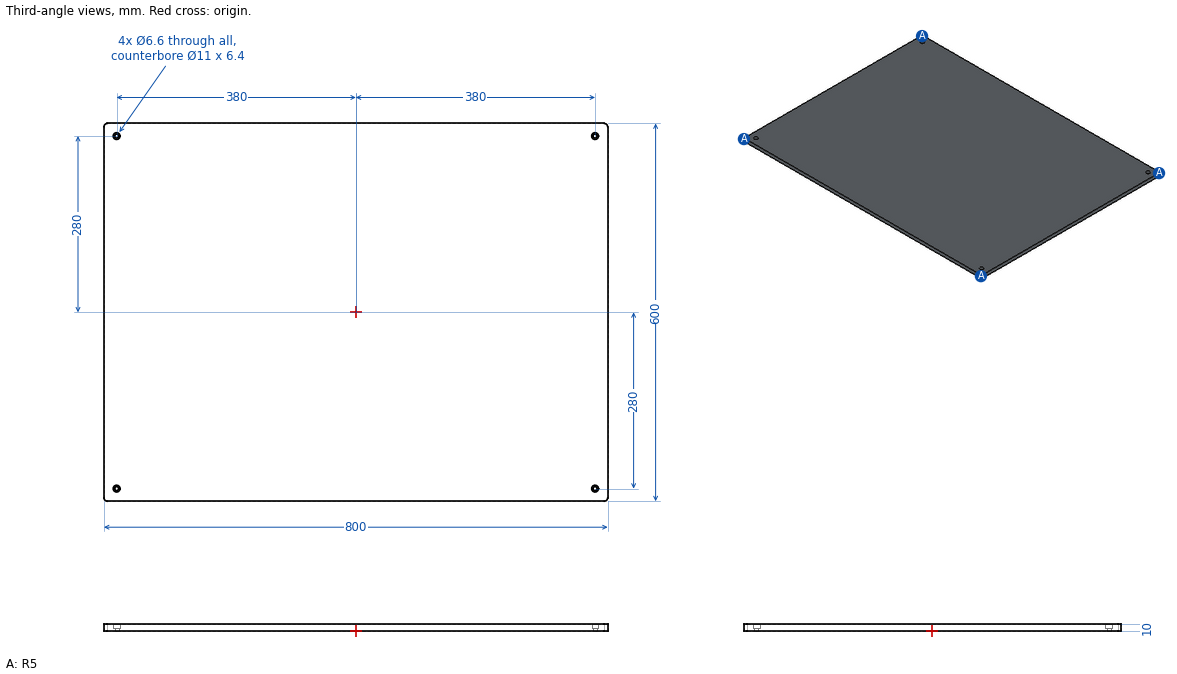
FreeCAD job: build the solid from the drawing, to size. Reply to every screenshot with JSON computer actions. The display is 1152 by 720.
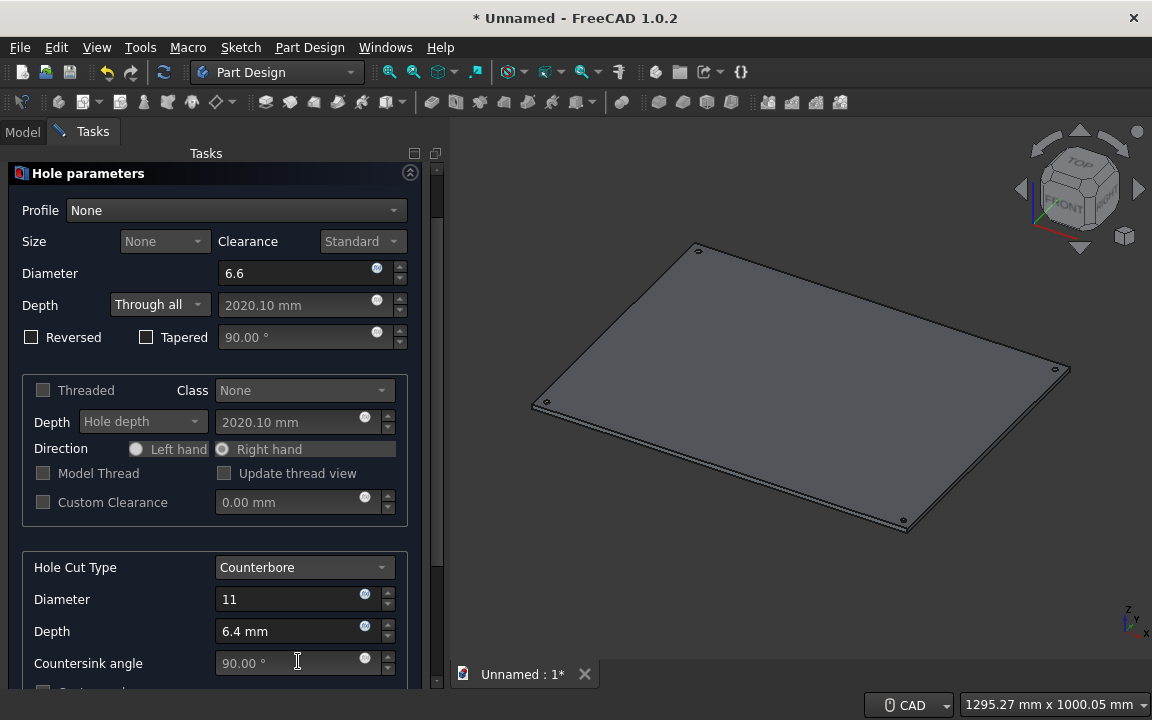
{"action": "scroll", "coordinate": [437, 426], "scroll_direction": "up", "scroll_amount": 2}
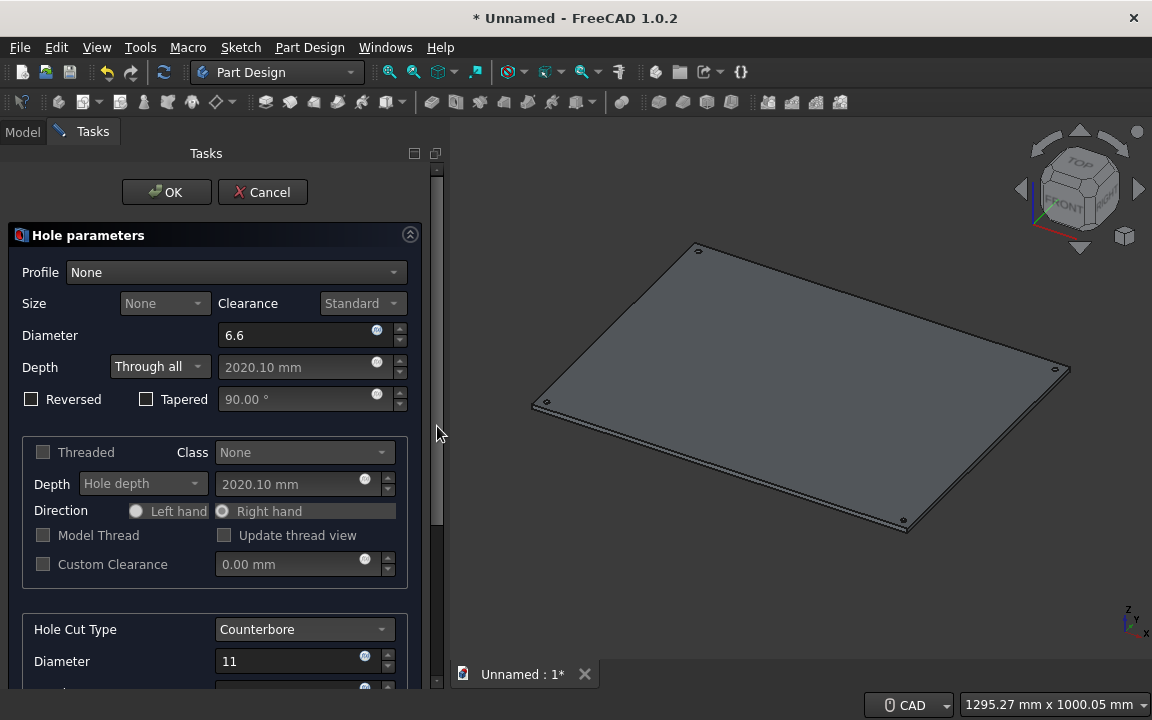
{"action": "left_click", "coordinate": [167, 192]}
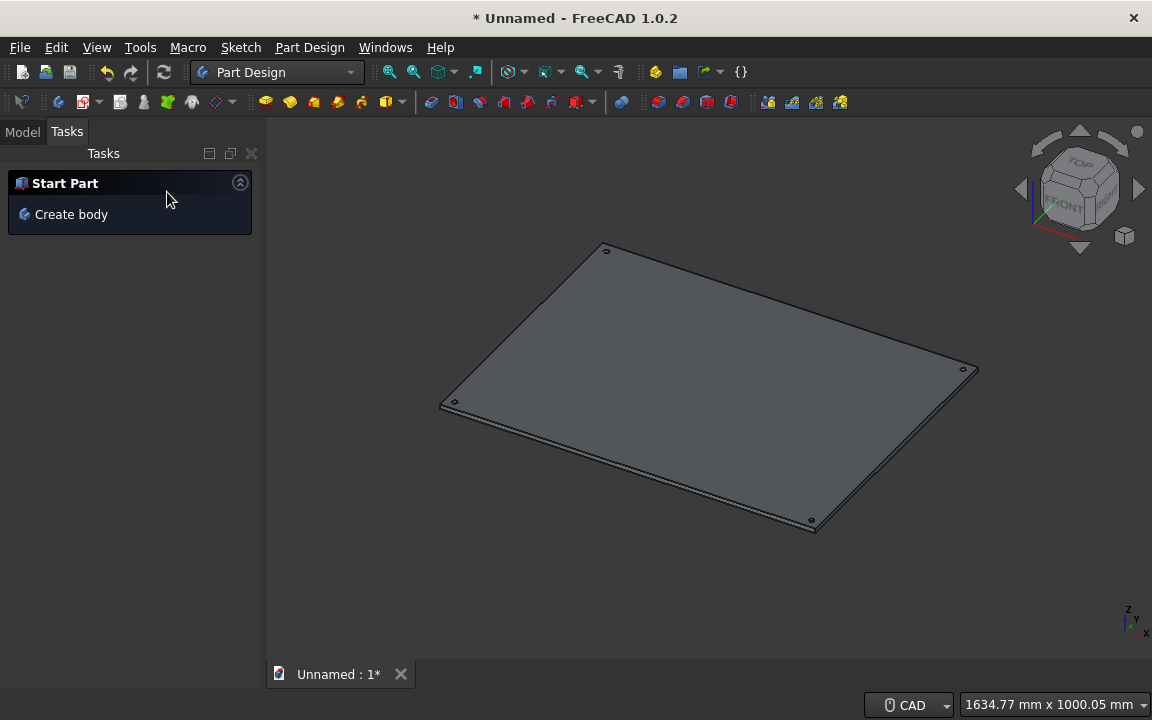
{"action": "scroll", "coordinate": [815, 530], "scroll_direction": "up", "scroll_amount": 10}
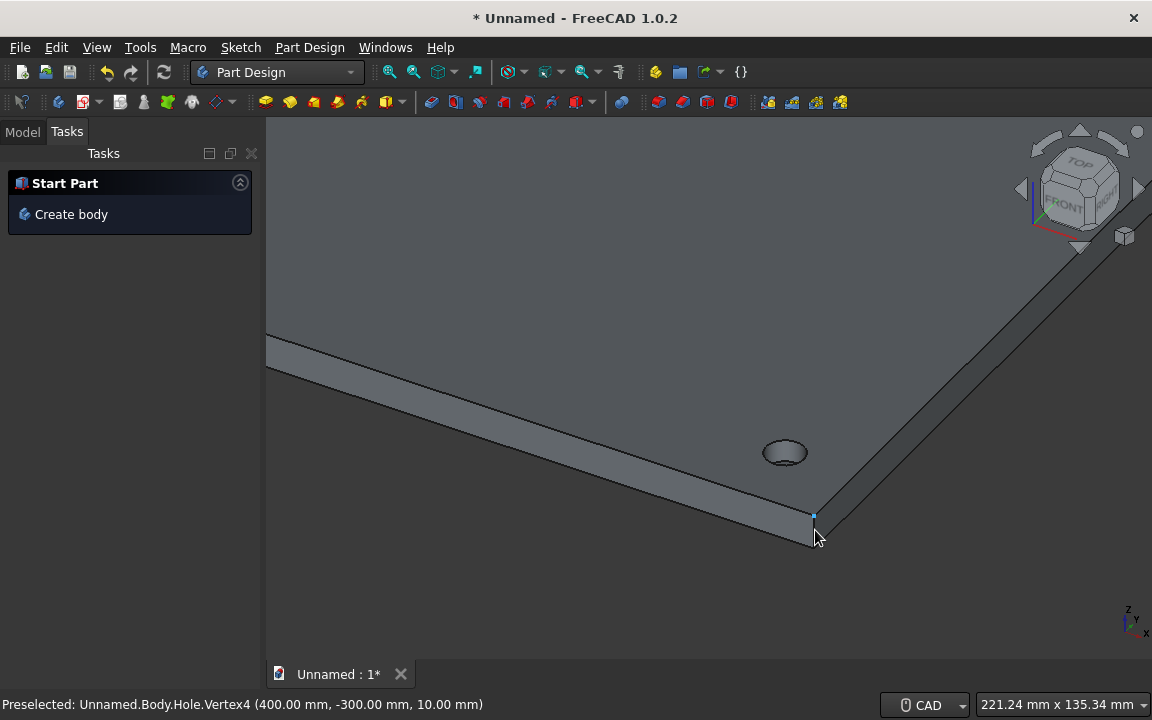
{"action": "left_click", "coordinate": [814, 531]}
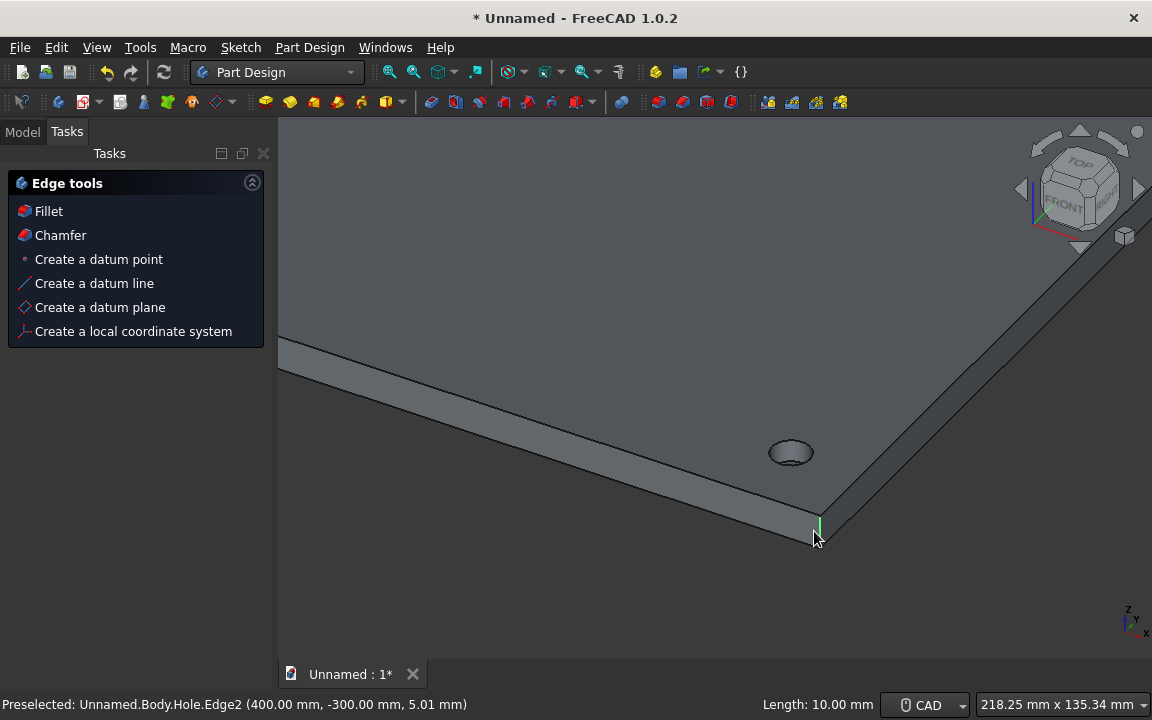
{"action": "left_click", "coordinate": [390, 72]}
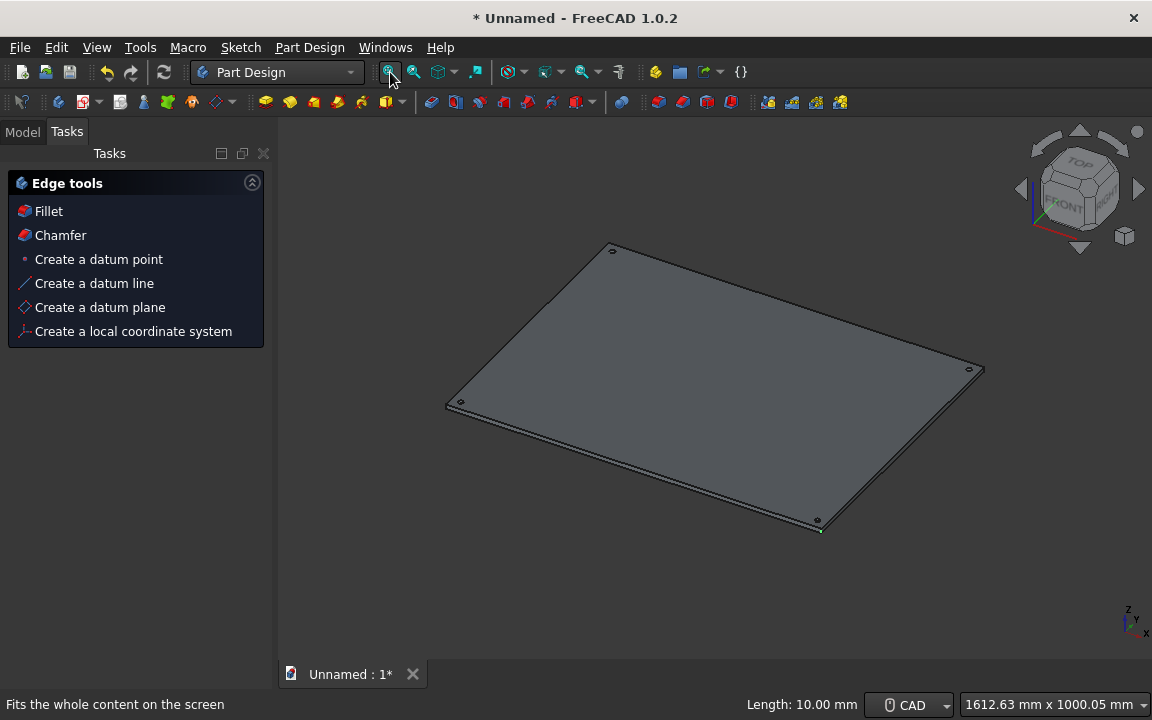
{"action": "key", "text": "0"}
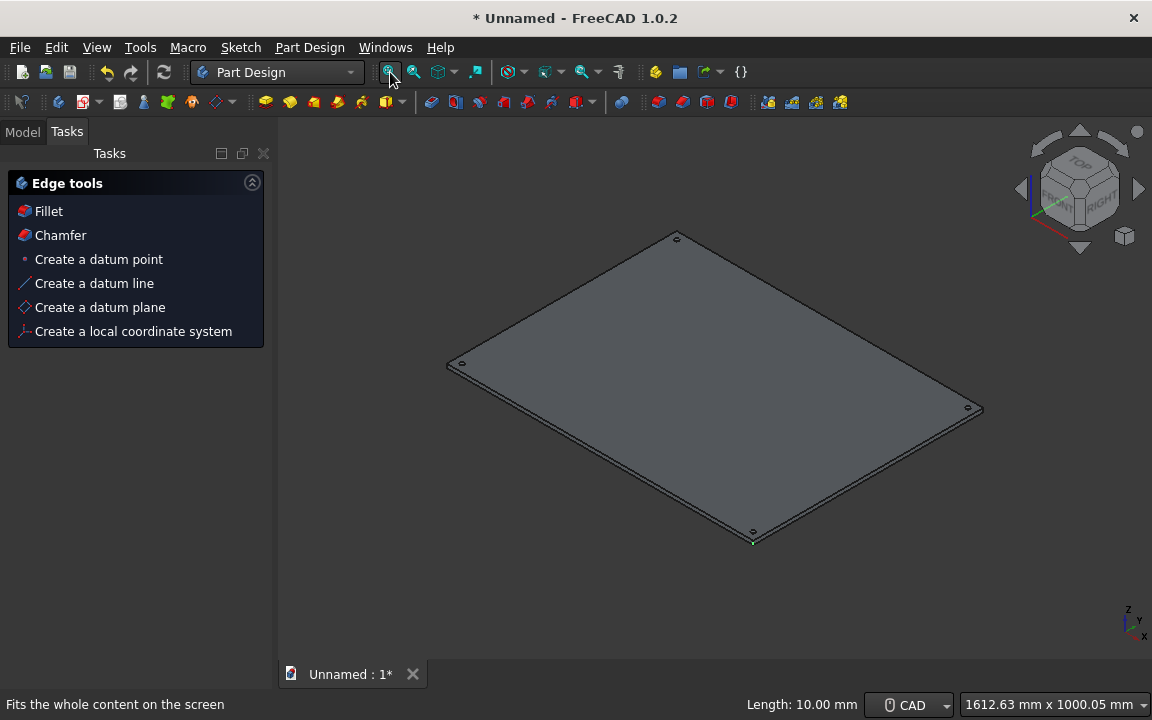
{"action": "scroll", "coordinate": [447, 365], "scroll_direction": "up", "scroll_amount": 10}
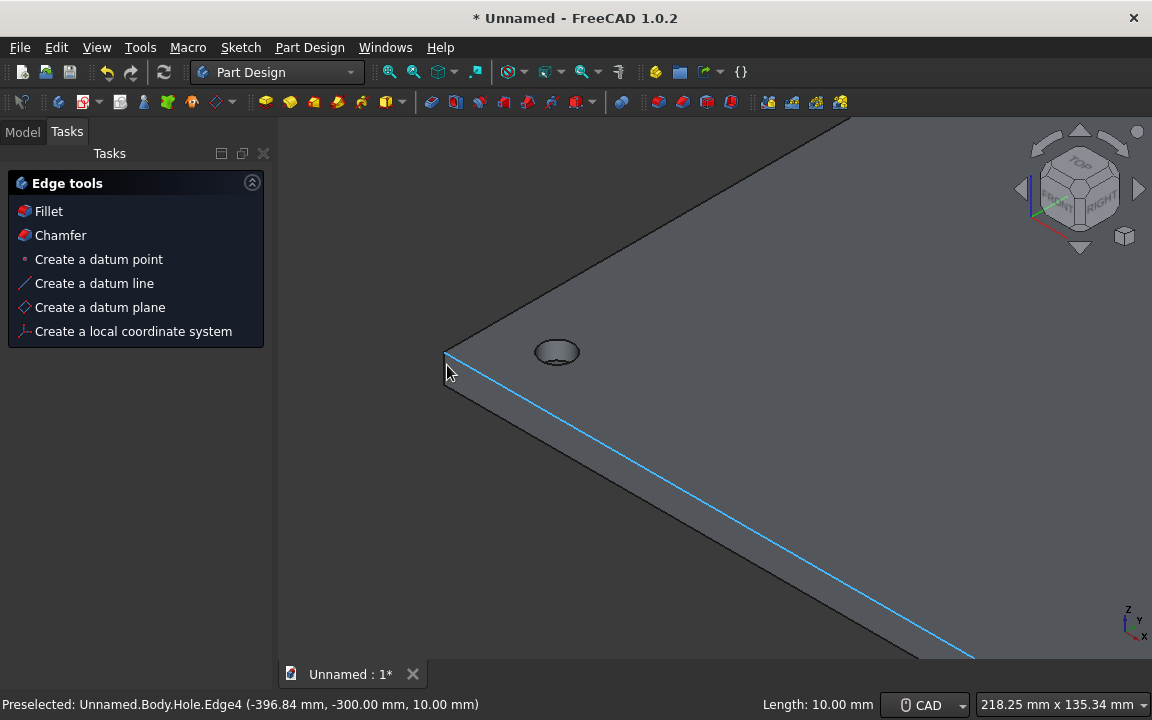
{"action": "key", "text": "v f"}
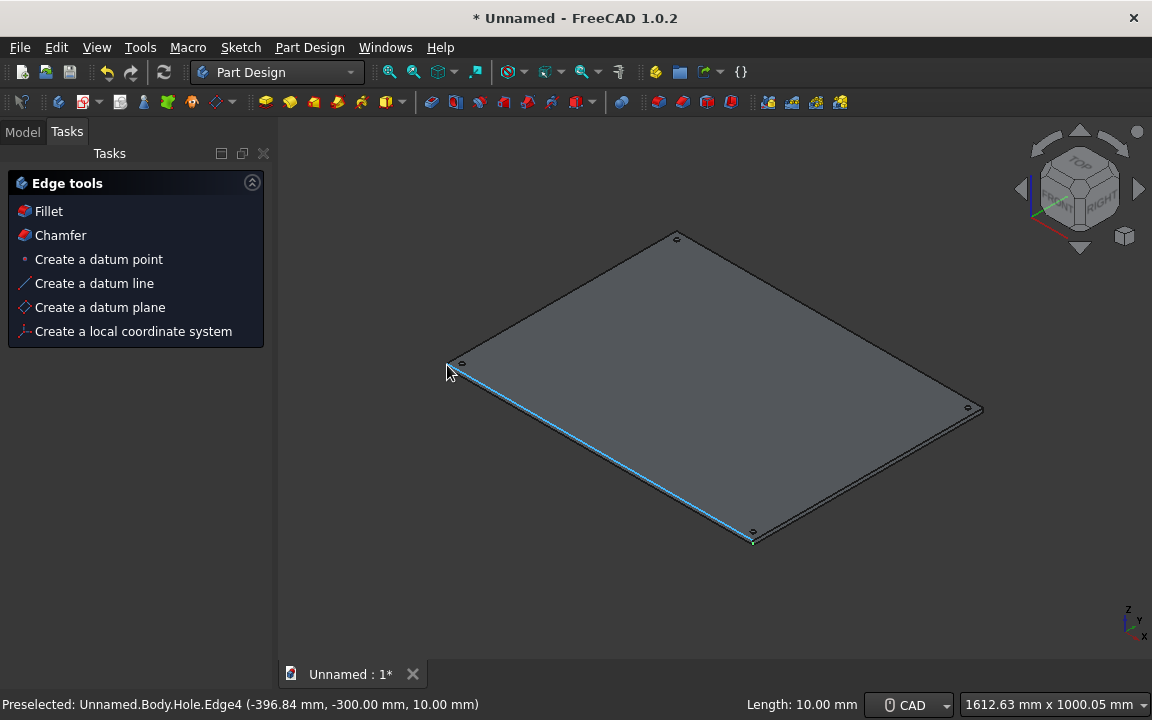
{"action": "key", "text": "2"}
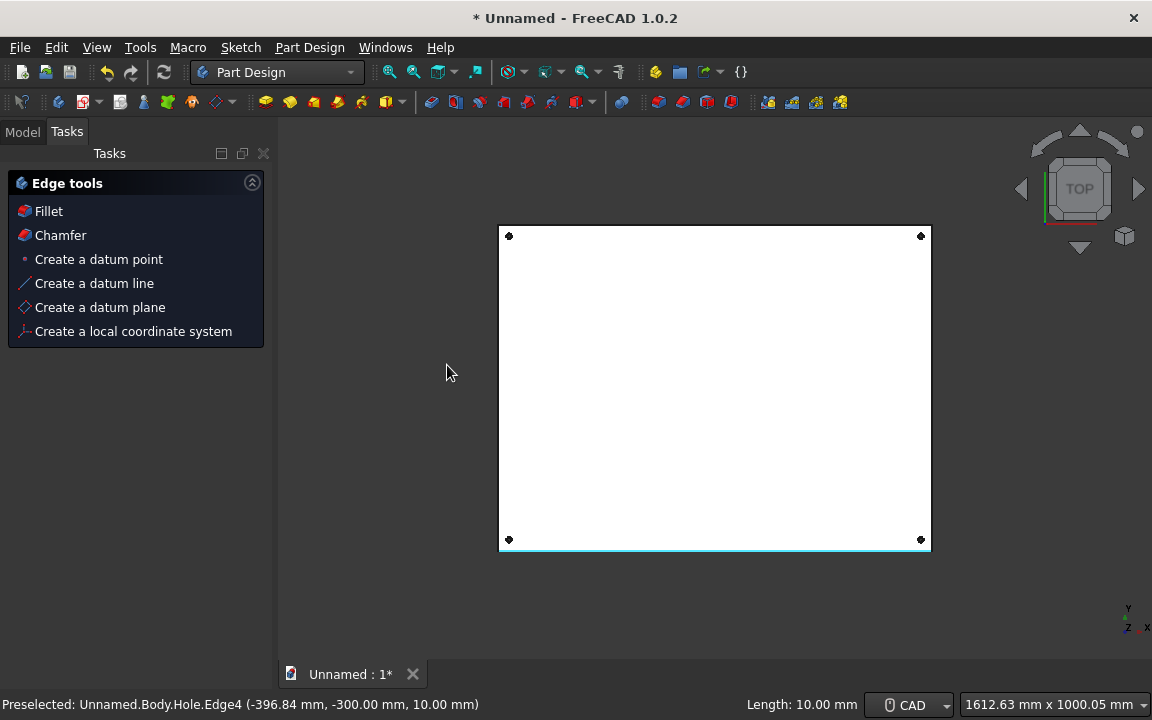
{"action": "scroll", "coordinate": [498, 550], "scroll_direction": "up", "scroll_amount": 10}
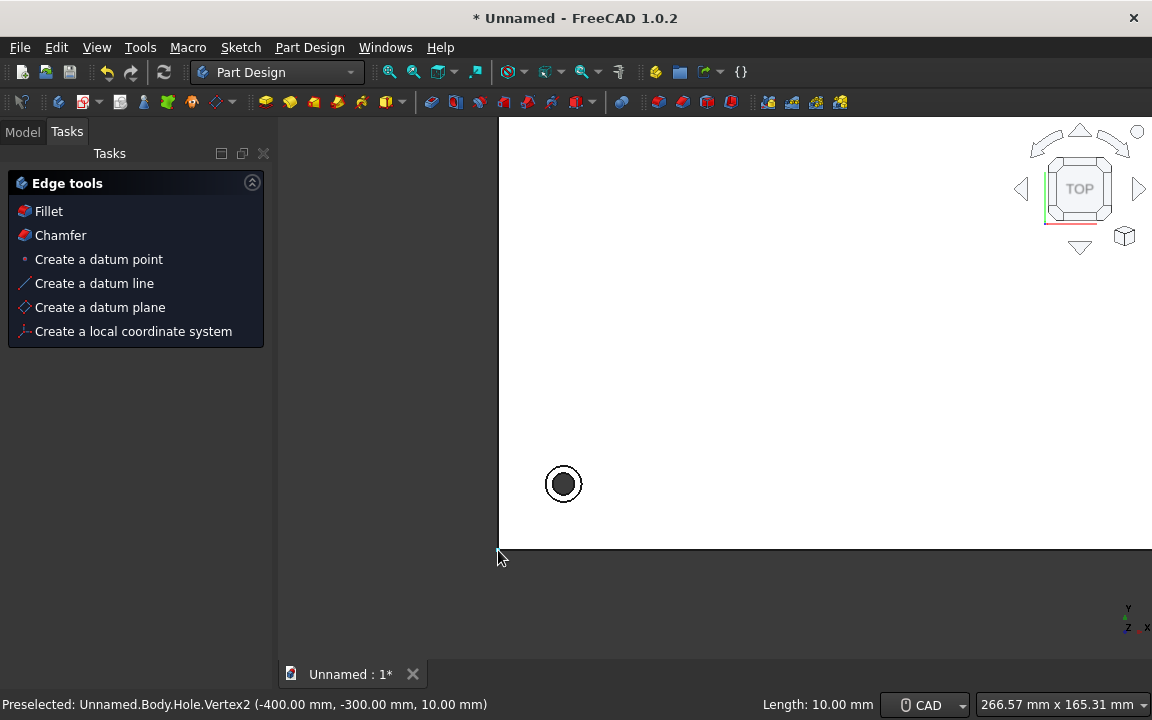
{"action": "key", "text": "v f"}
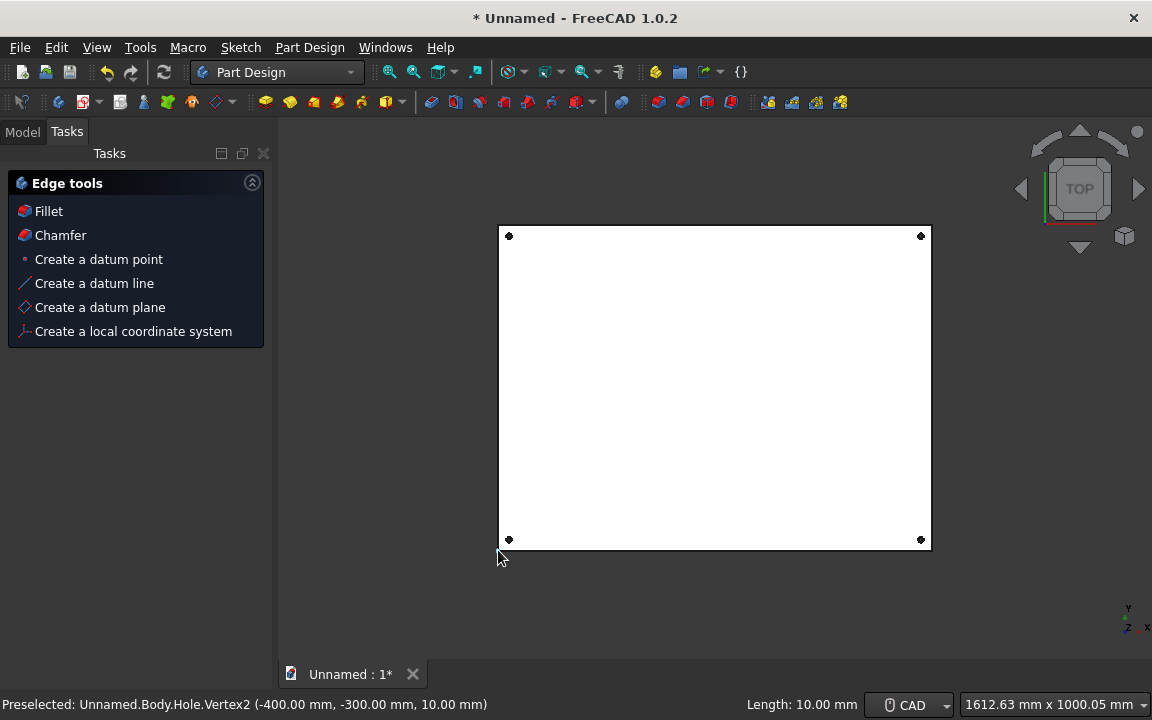
{"action": "key", "text": "1"}